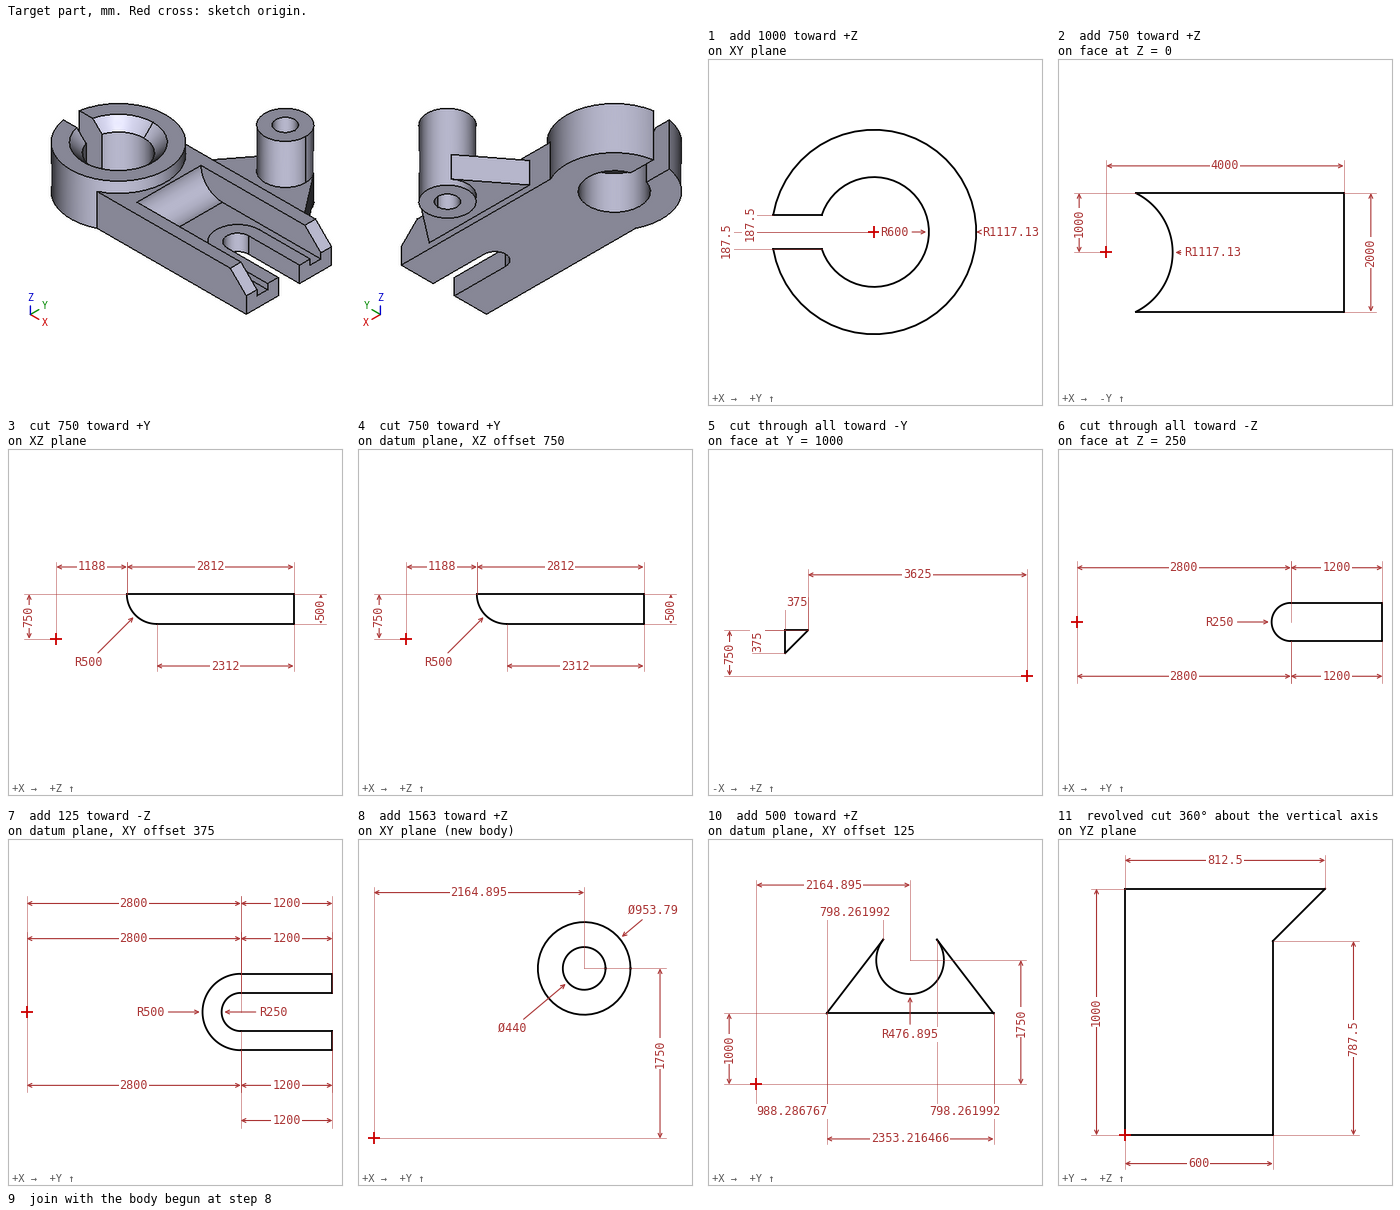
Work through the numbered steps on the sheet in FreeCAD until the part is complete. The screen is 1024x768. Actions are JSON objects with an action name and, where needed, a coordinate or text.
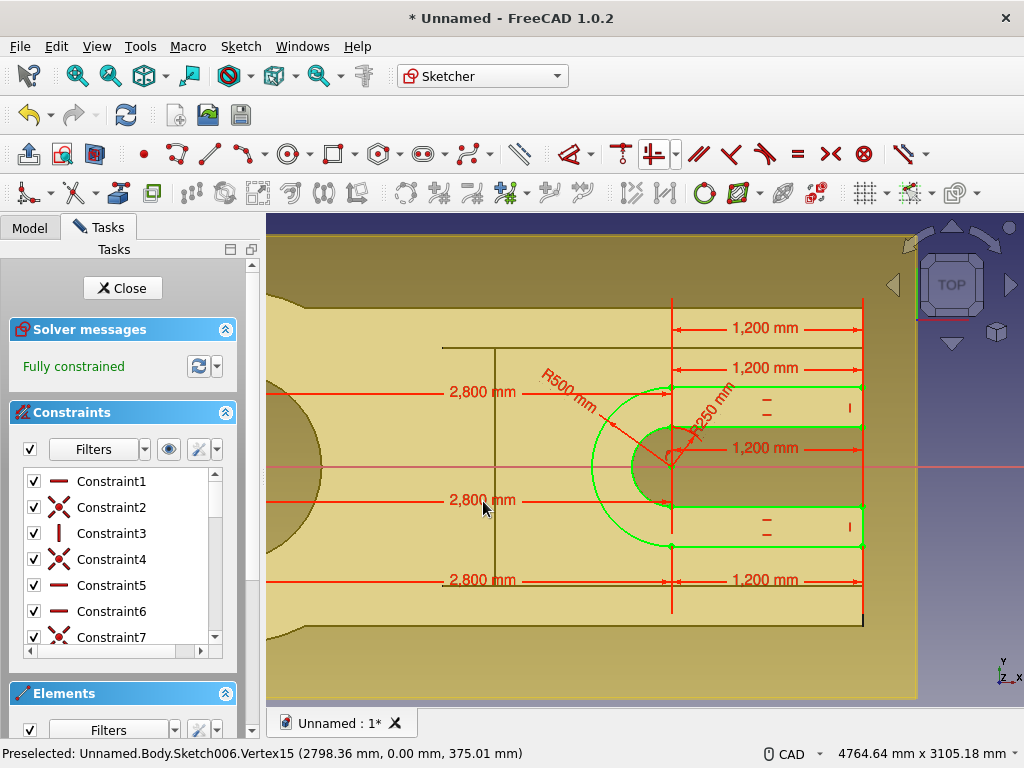
{"action": "left_click", "coordinate": [123, 288]}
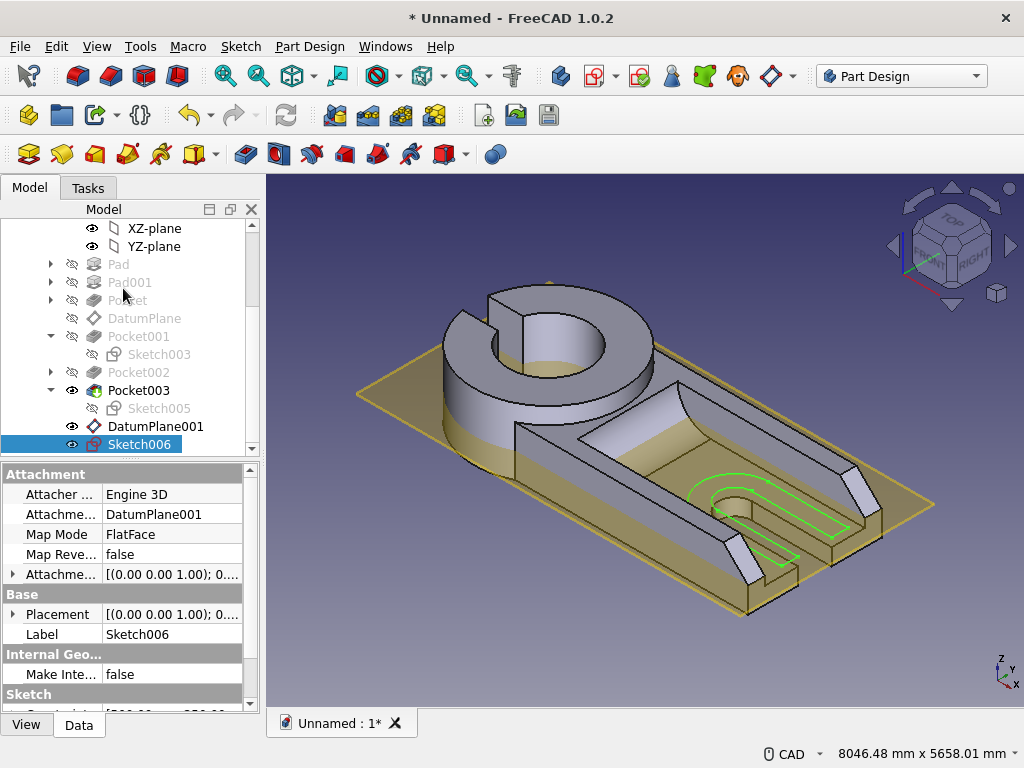
{"action": "left_click", "coordinate": [29, 154]}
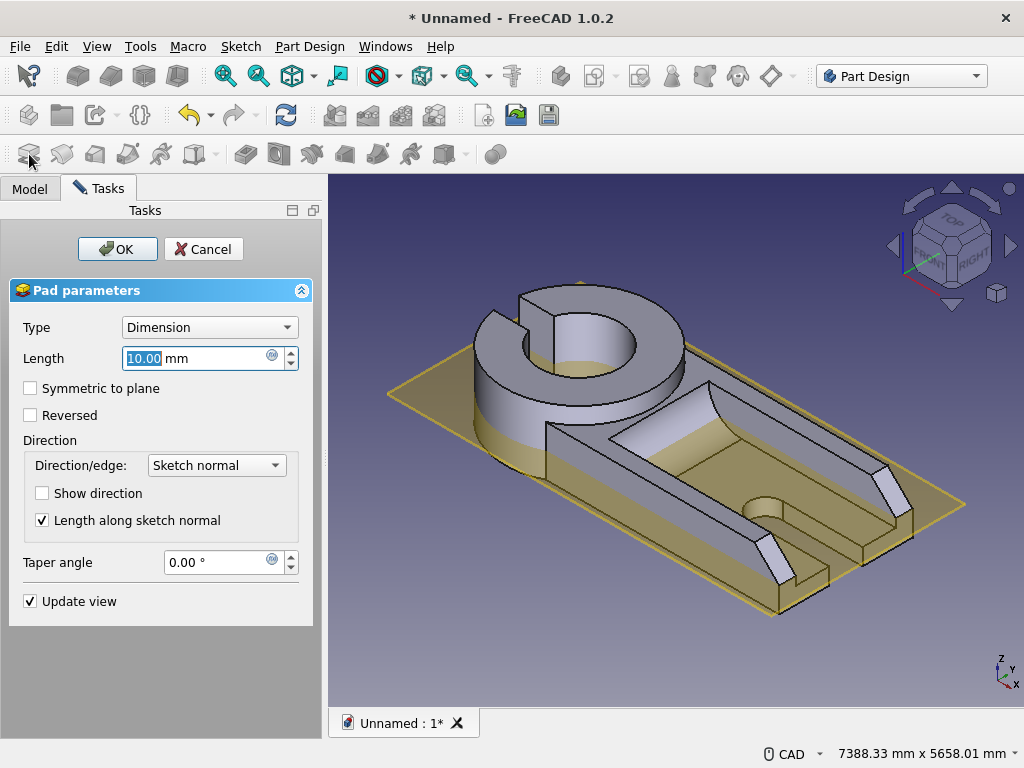
{"action": "type", "text": "125"}
{"action": "key", "text": "Tab"}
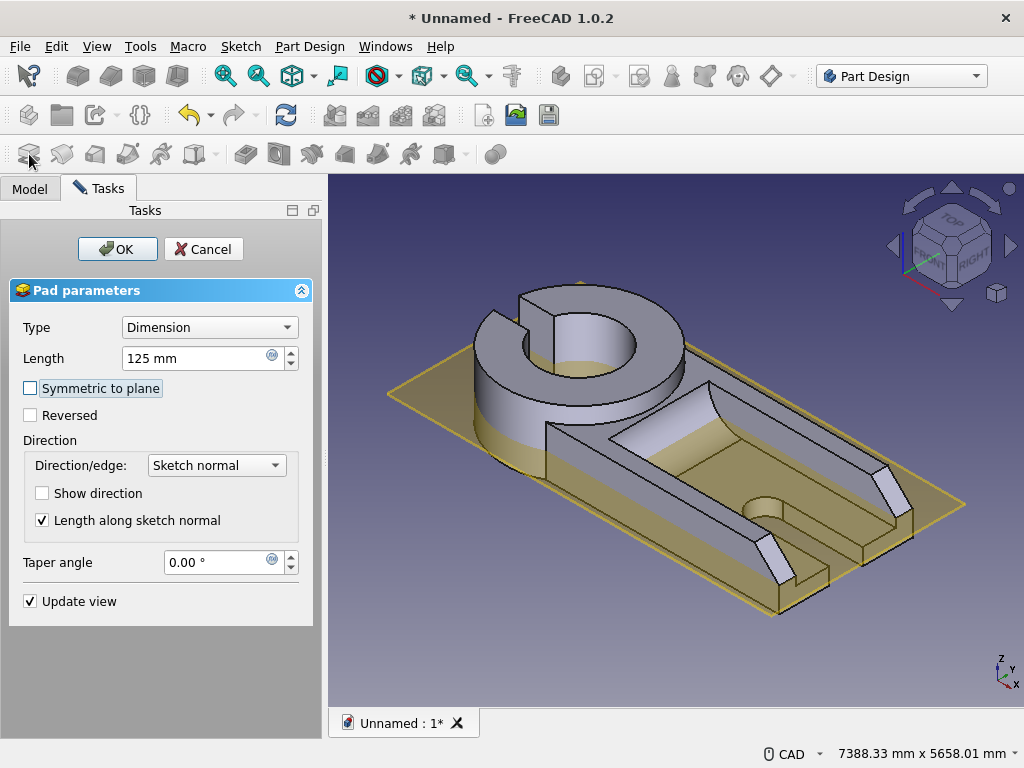
{"action": "left_click", "coordinate": [31, 415]}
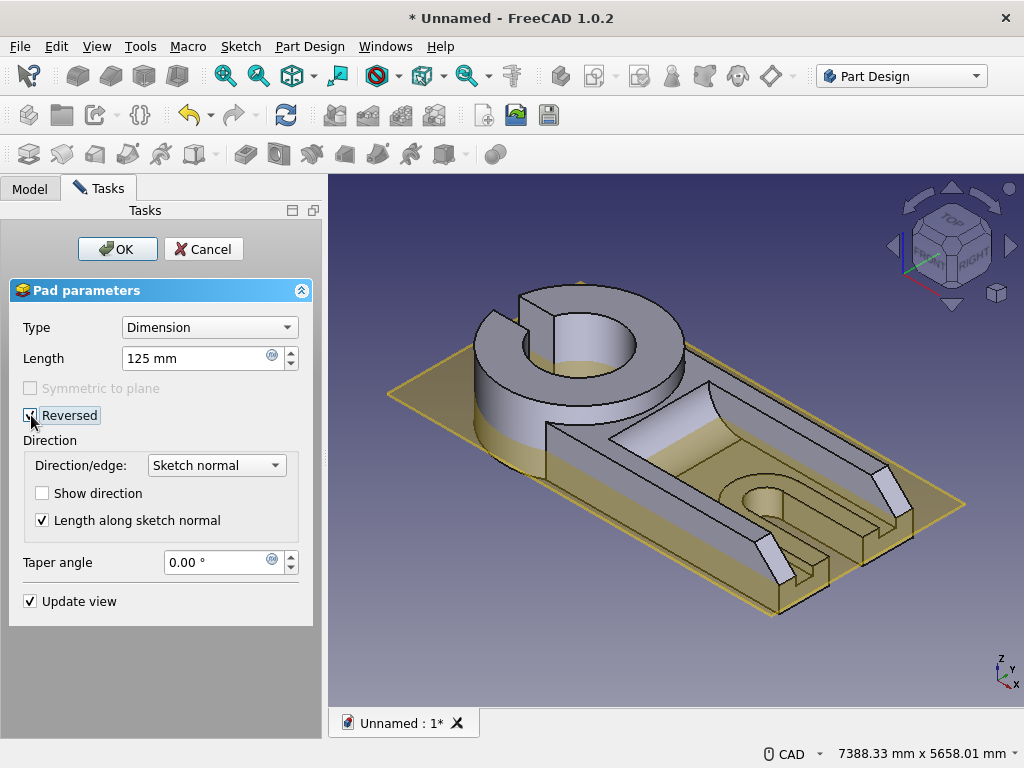
{"action": "left_click", "coordinate": [118, 249]}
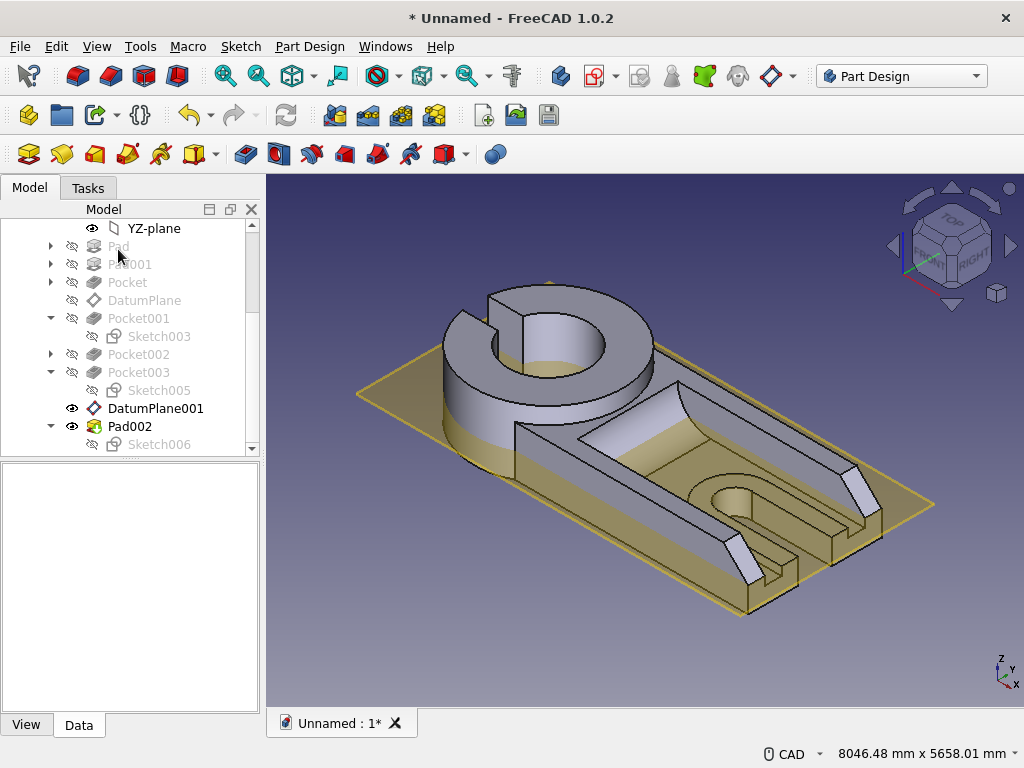
{"action": "left_click", "coordinate": [117, 408]}
{"action": "key", "text": "space"}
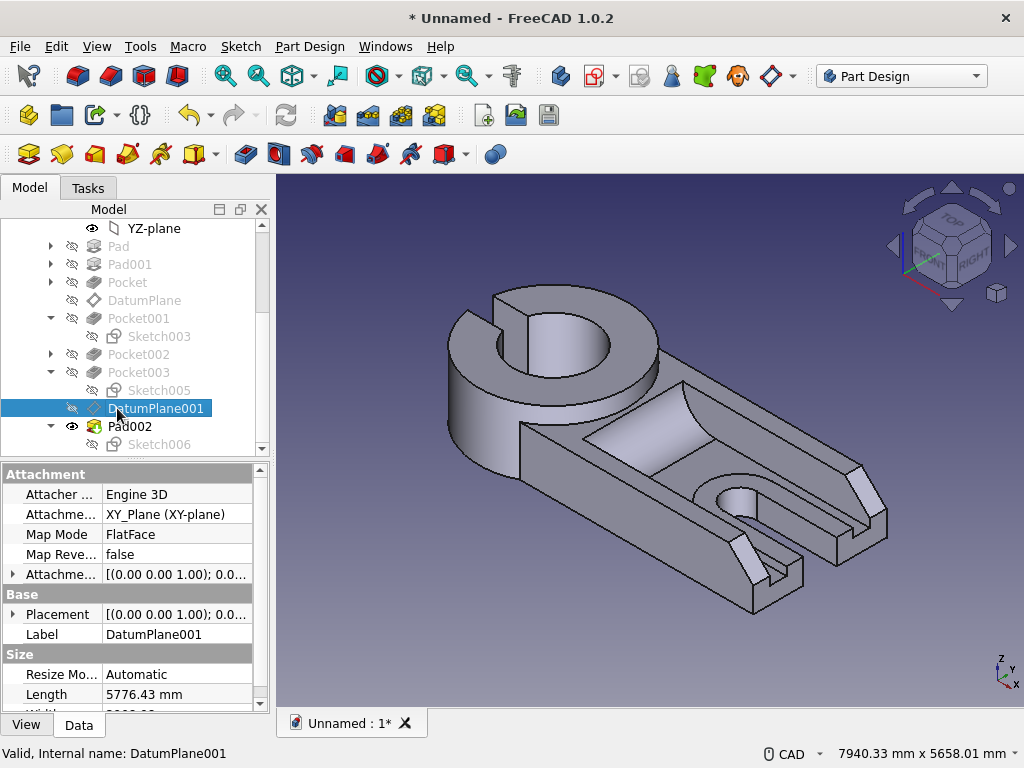
{"action": "left_click", "coordinate": [316, 667]}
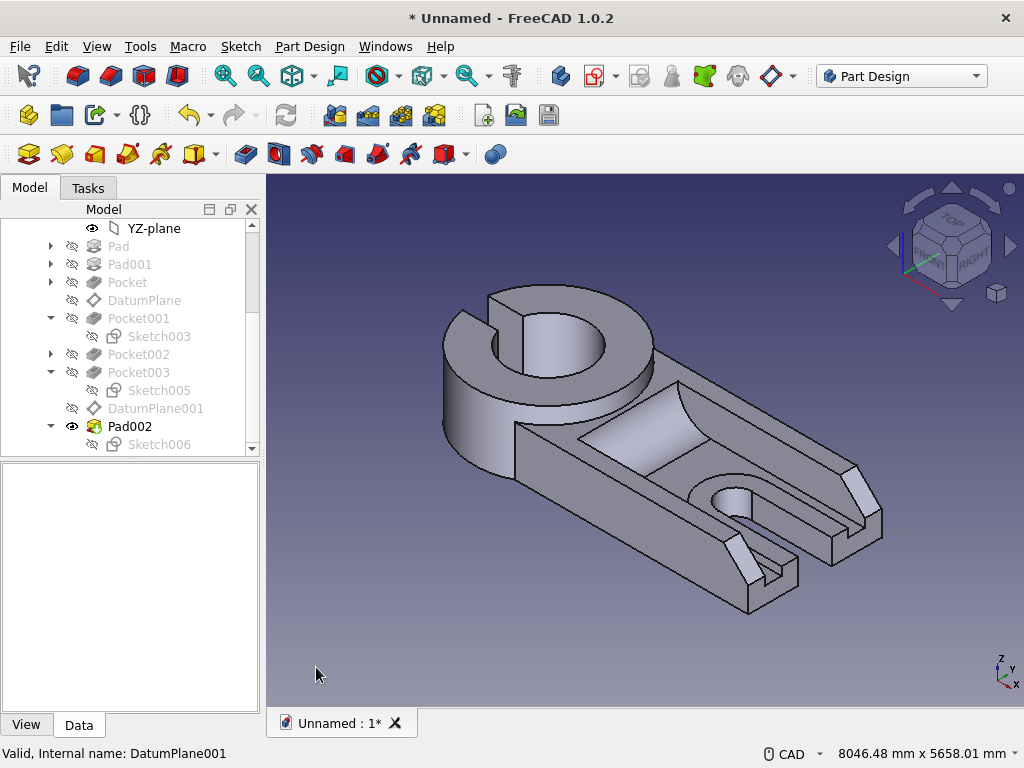
{"action": "left_click", "coordinate": [561, 76]}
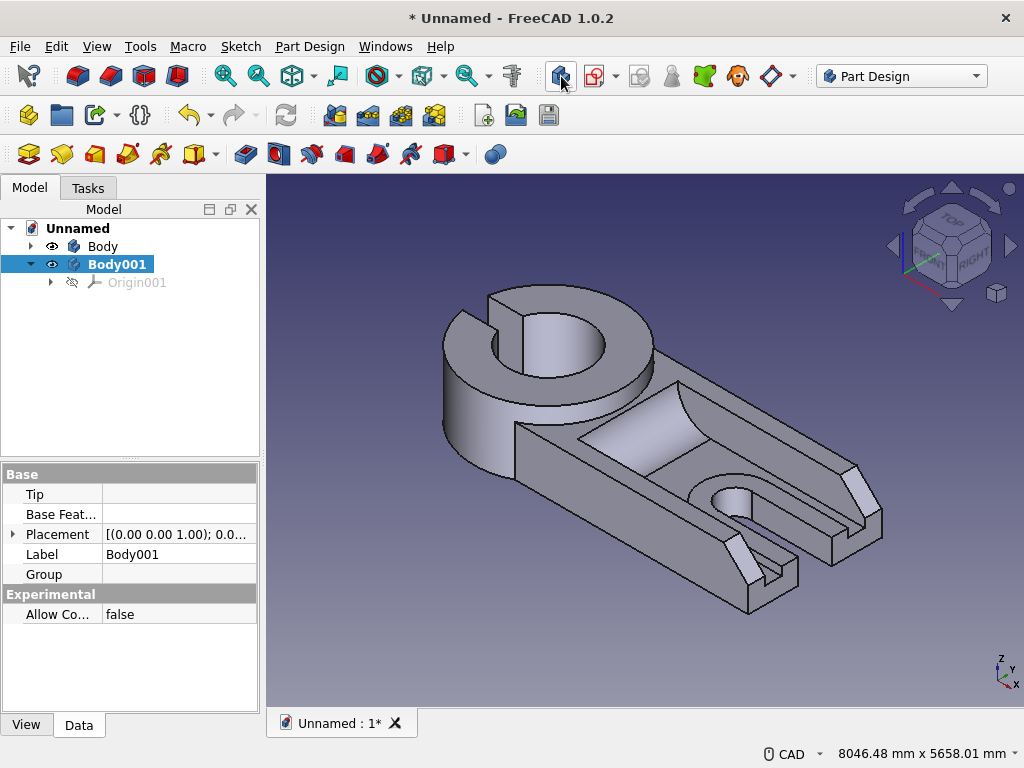
{"action": "left_click", "coordinate": [306, 667]}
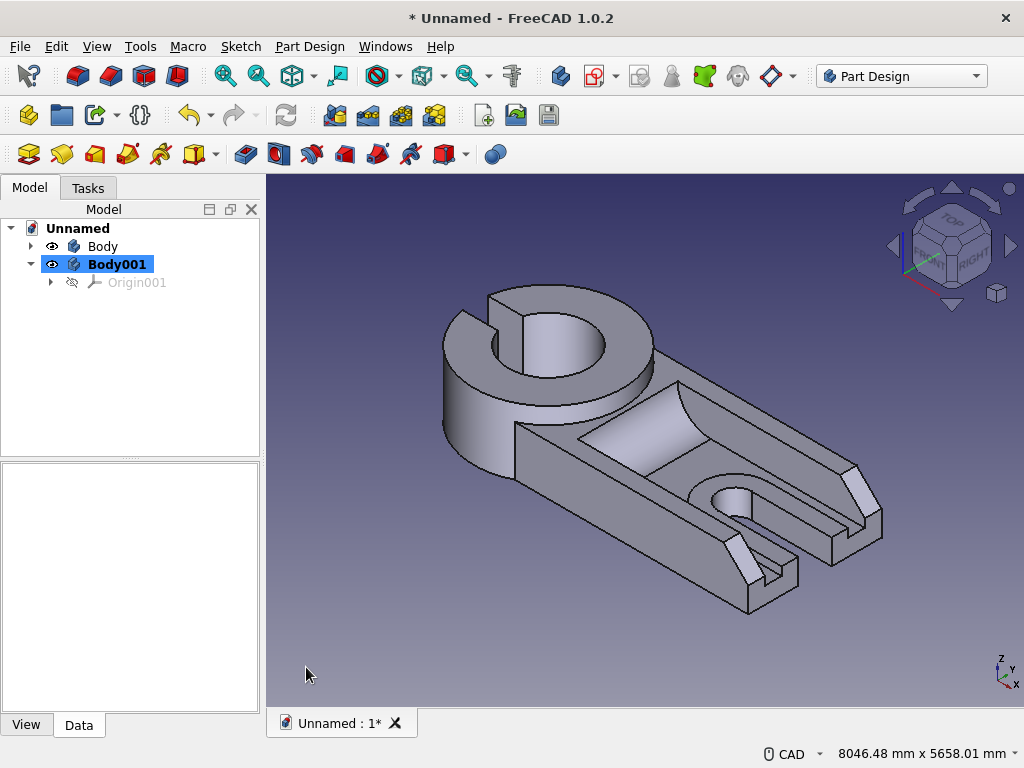
{"action": "left_click", "coordinate": [594, 76]}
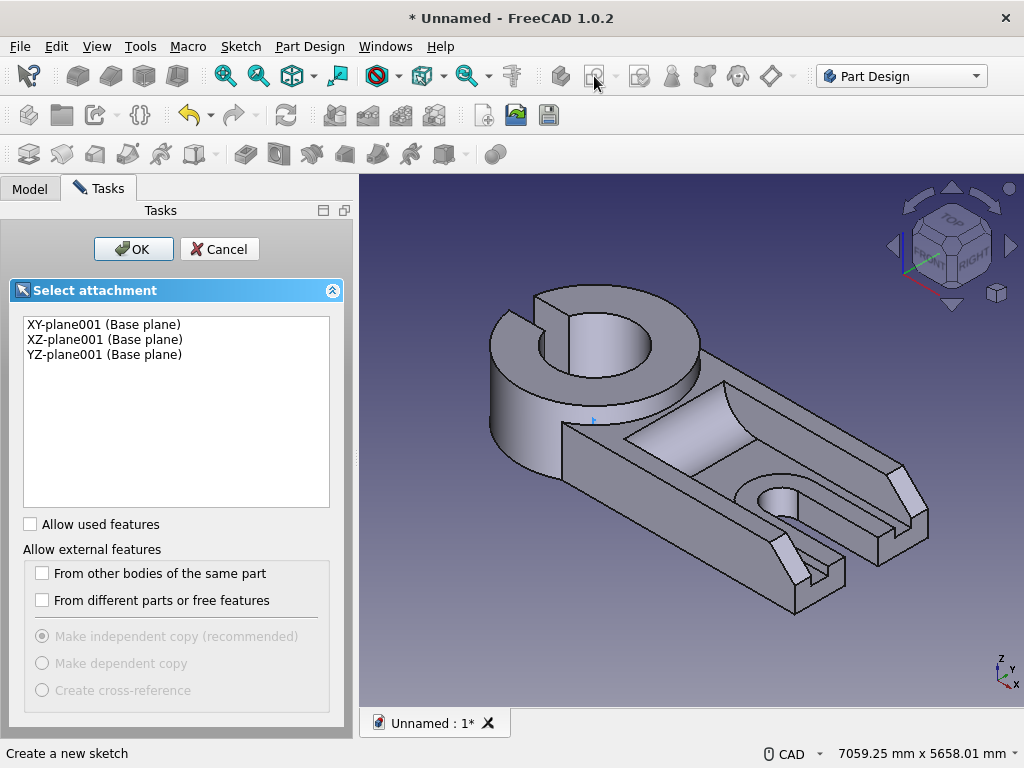
{"action": "left_click", "coordinate": [84, 324]}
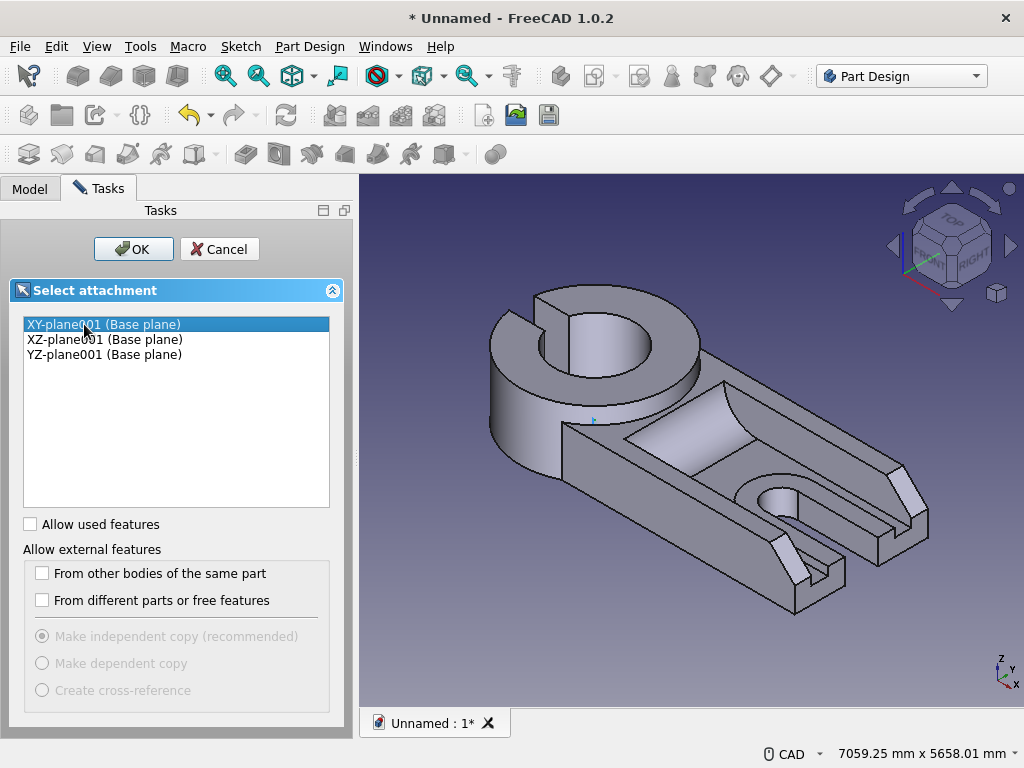
{"action": "left_click", "coordinate": [134, 249]}